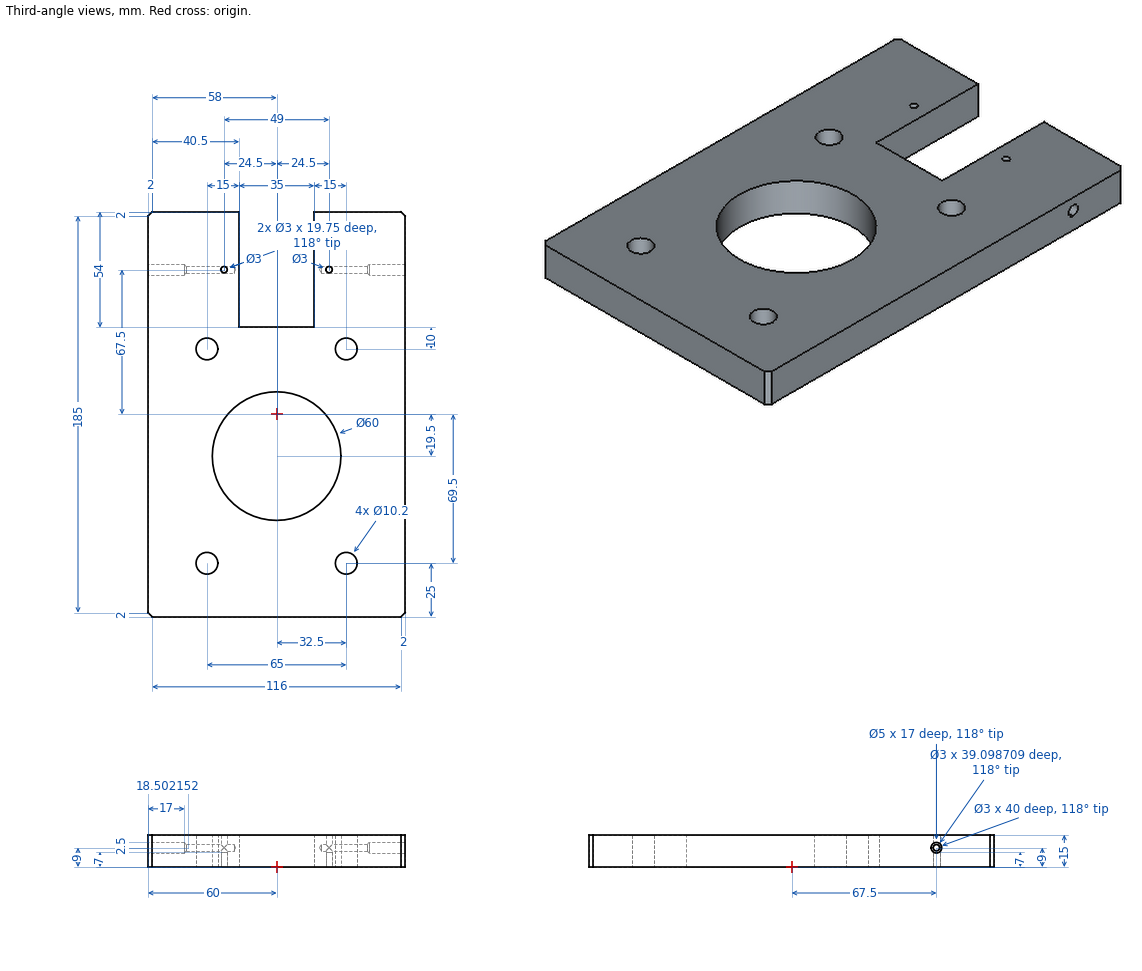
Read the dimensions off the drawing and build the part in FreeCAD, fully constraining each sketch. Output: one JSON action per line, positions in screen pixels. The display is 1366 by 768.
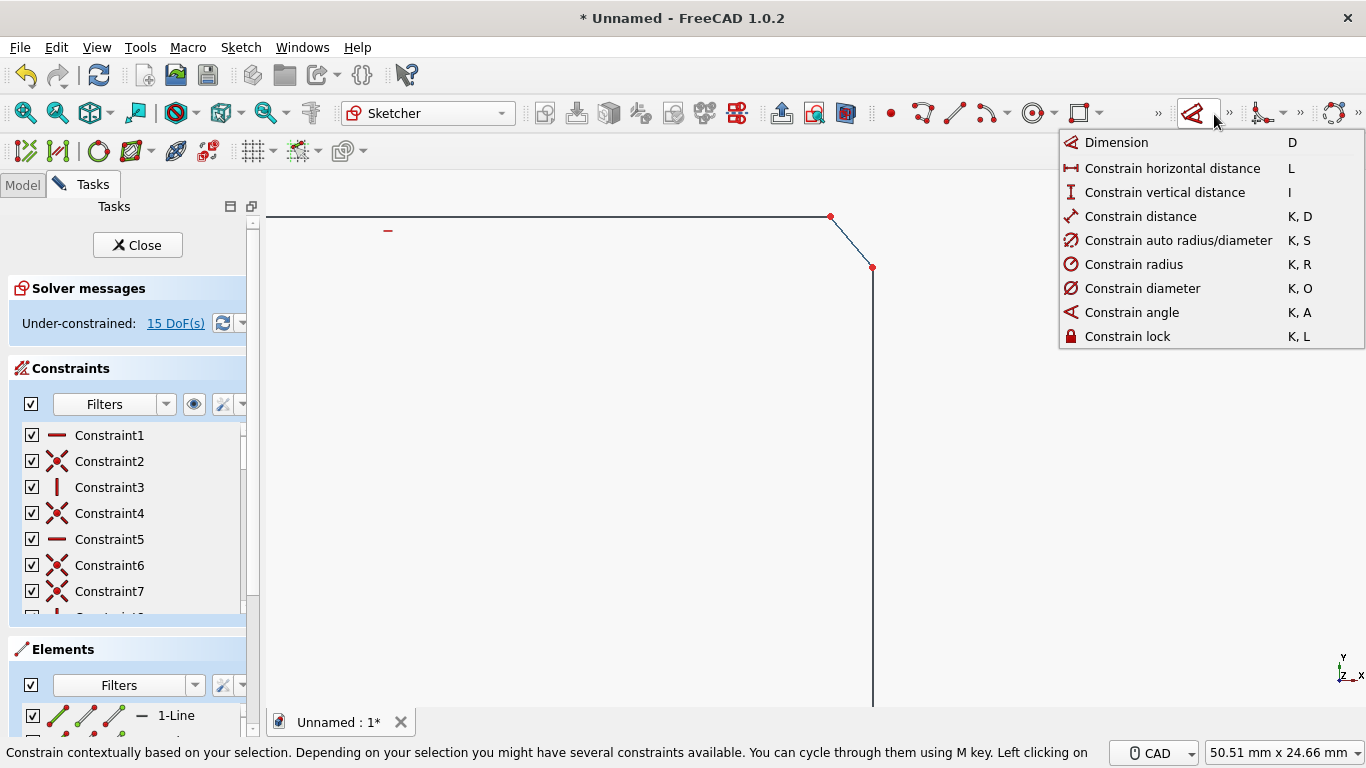
{"action": "left_click", "coordinate": [1212, 168]}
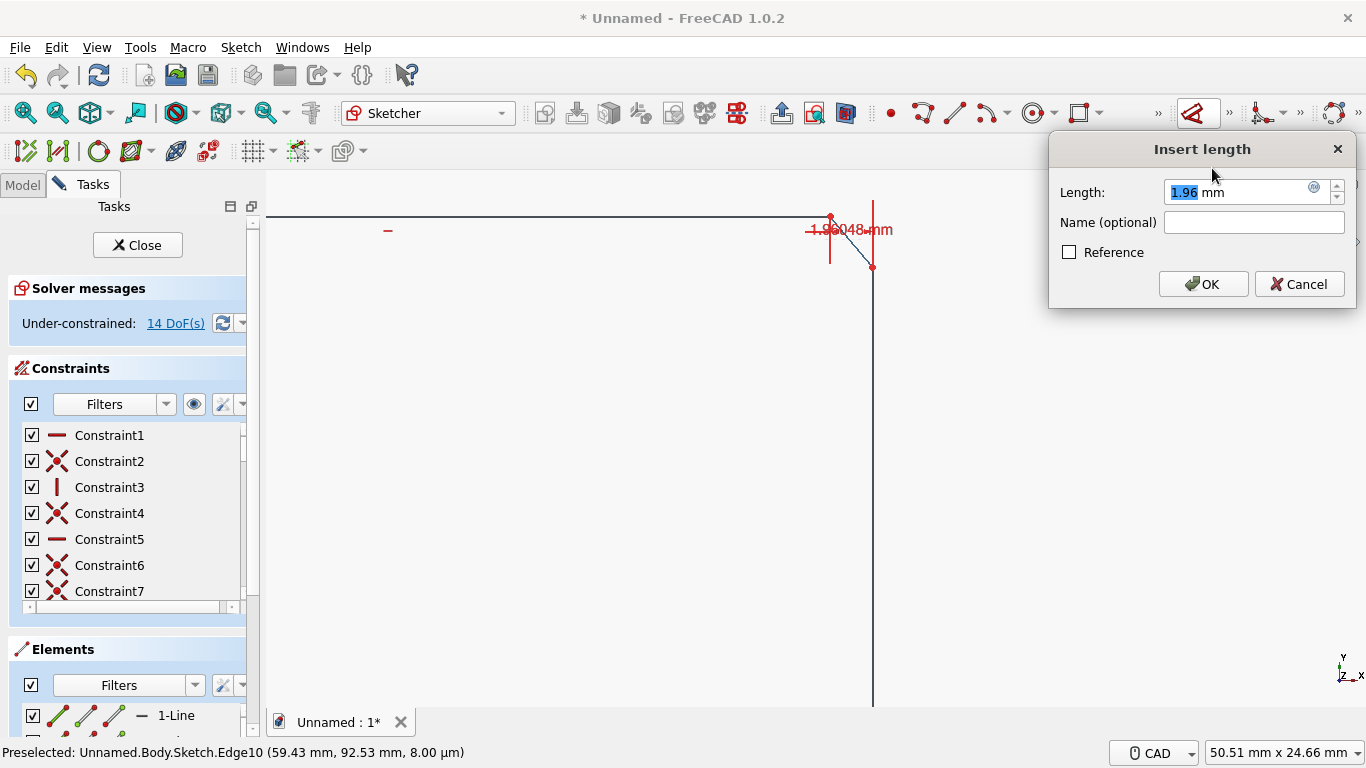
{"action": "type", "text": "2"}
{"action": "key", "text": "Return"}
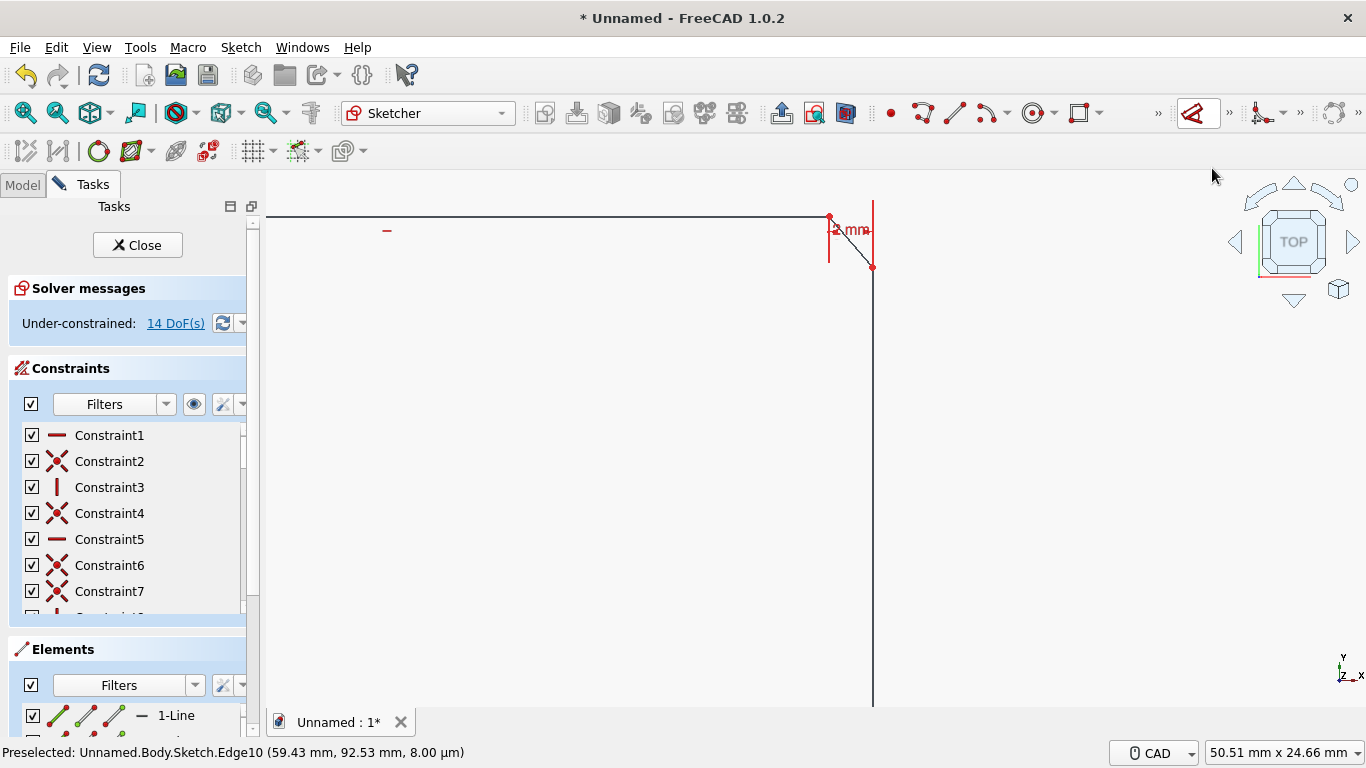
{"action": "left_click", "coordinate": [860, 252]}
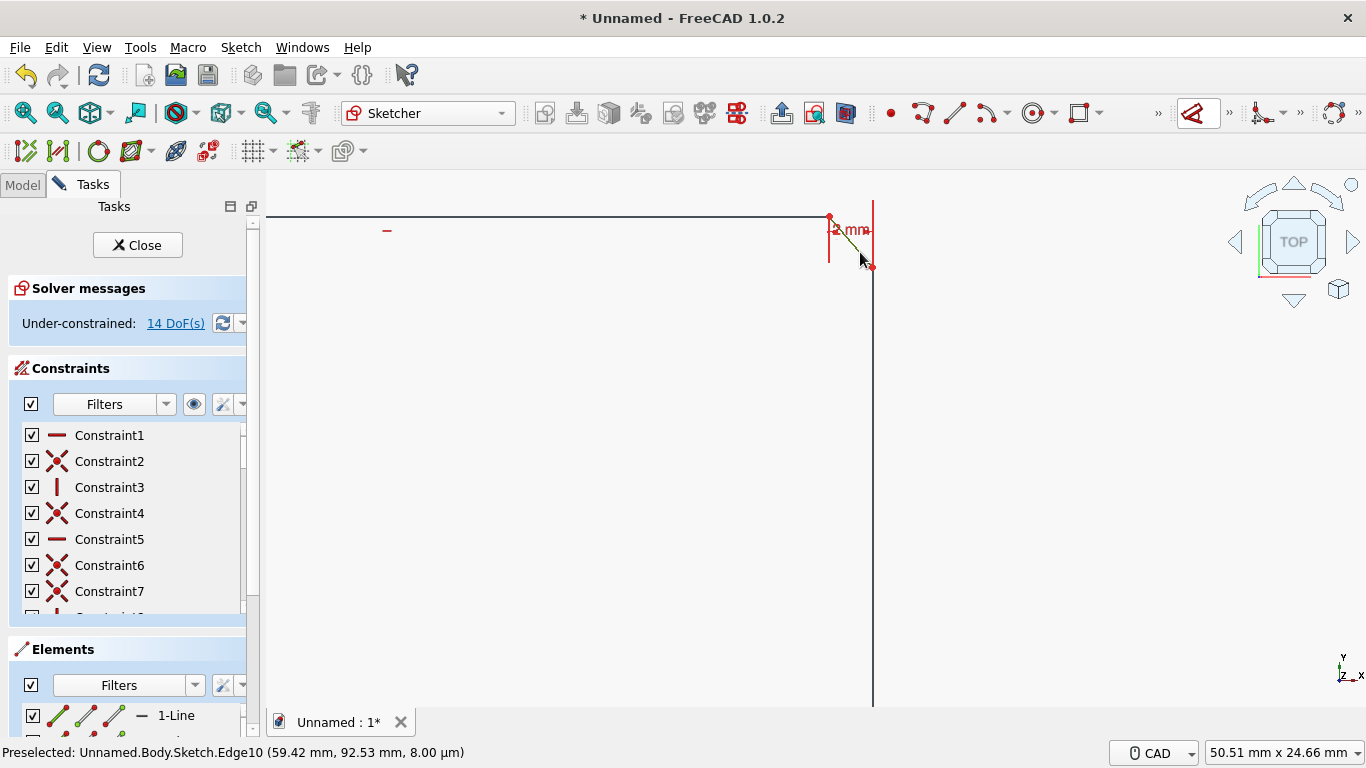
{"action": "left_click", "coordinate": [1214, 114]}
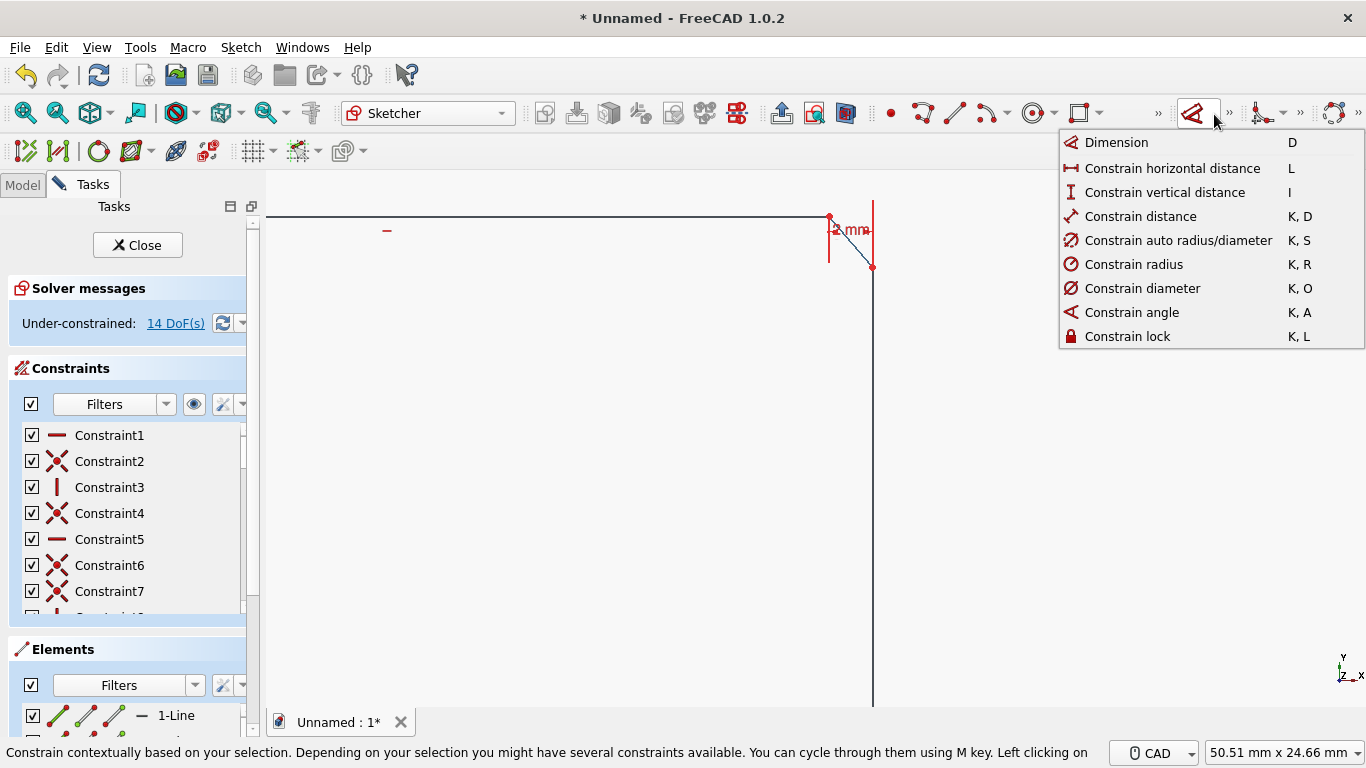
{"action": "left_click", "coordinate": [1212, 192]}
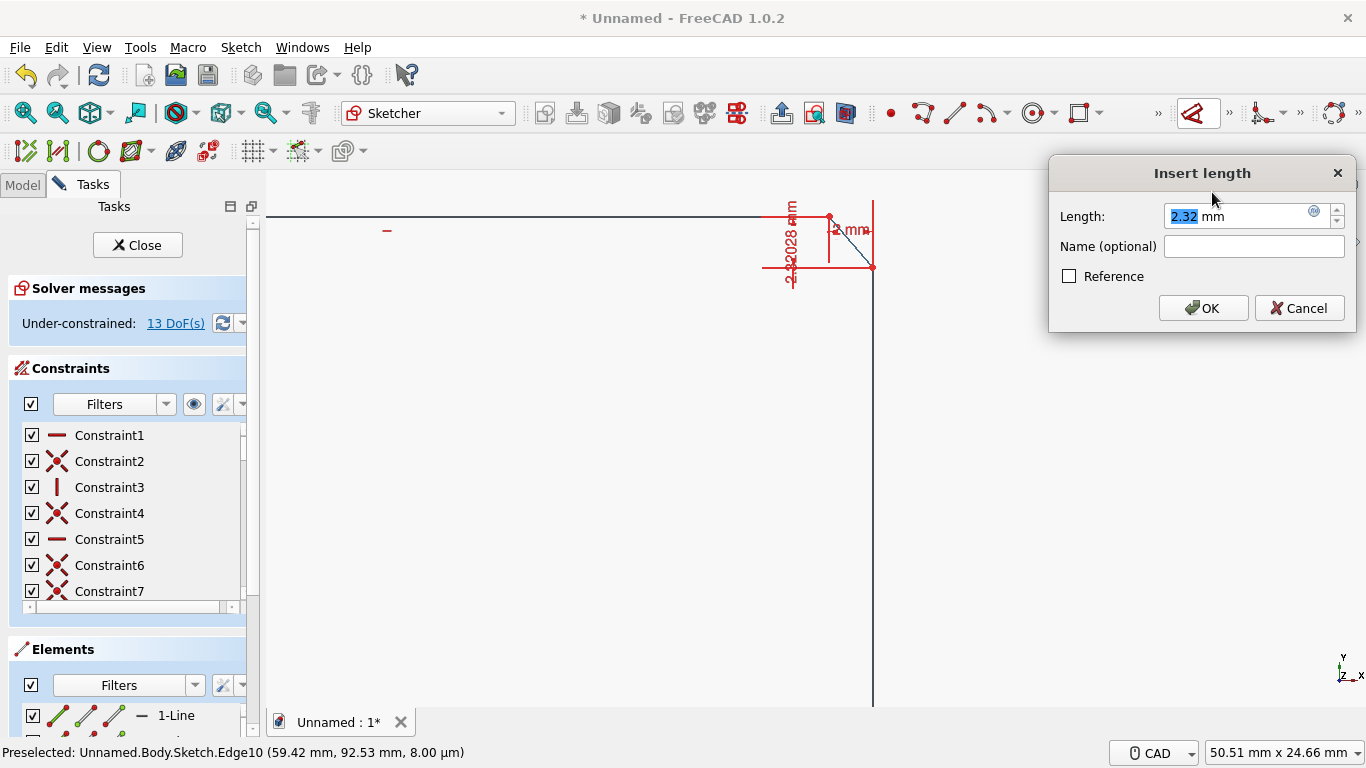
{"action": "type", "text": "2"}
{"action": "key", "text": "Return"}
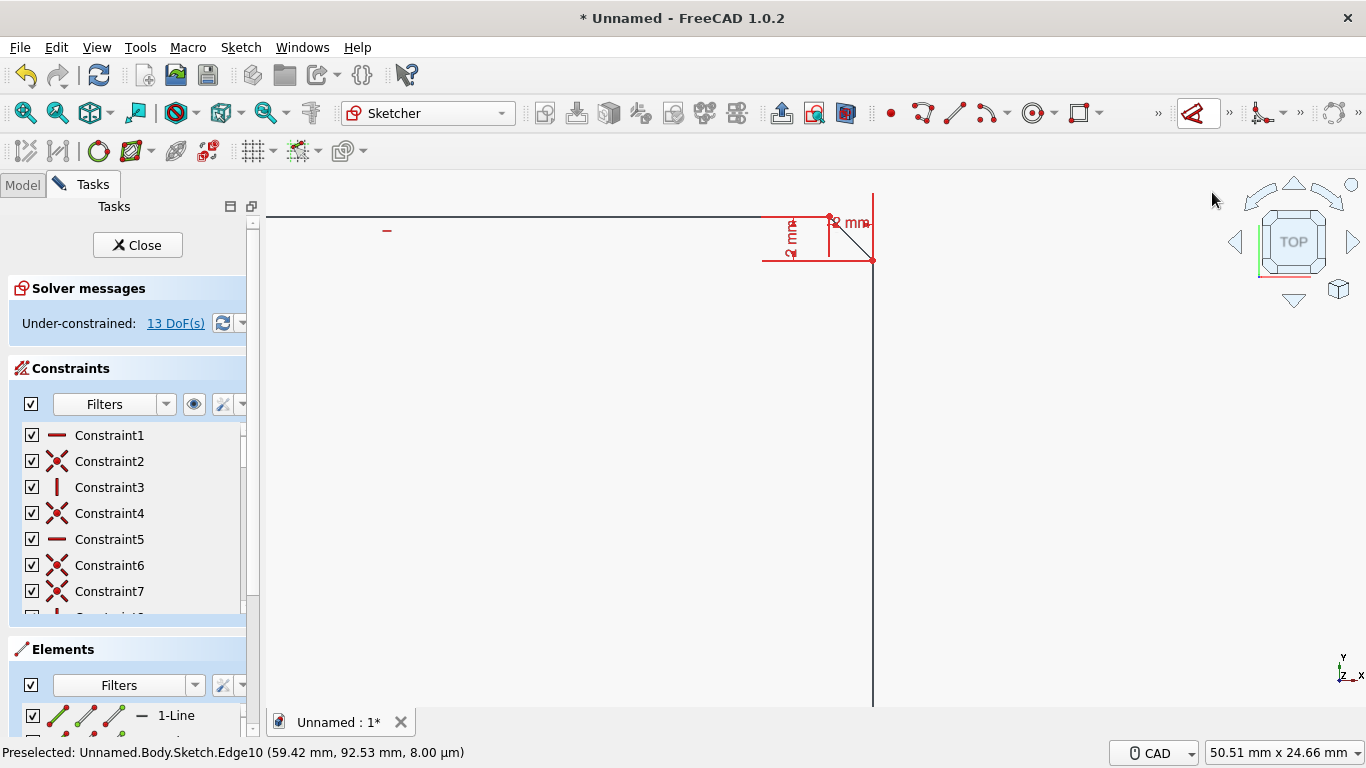
{"action": "scroll", "coordinate": [865, 256], "scroll_direction": "down", "scroll_amount": 12}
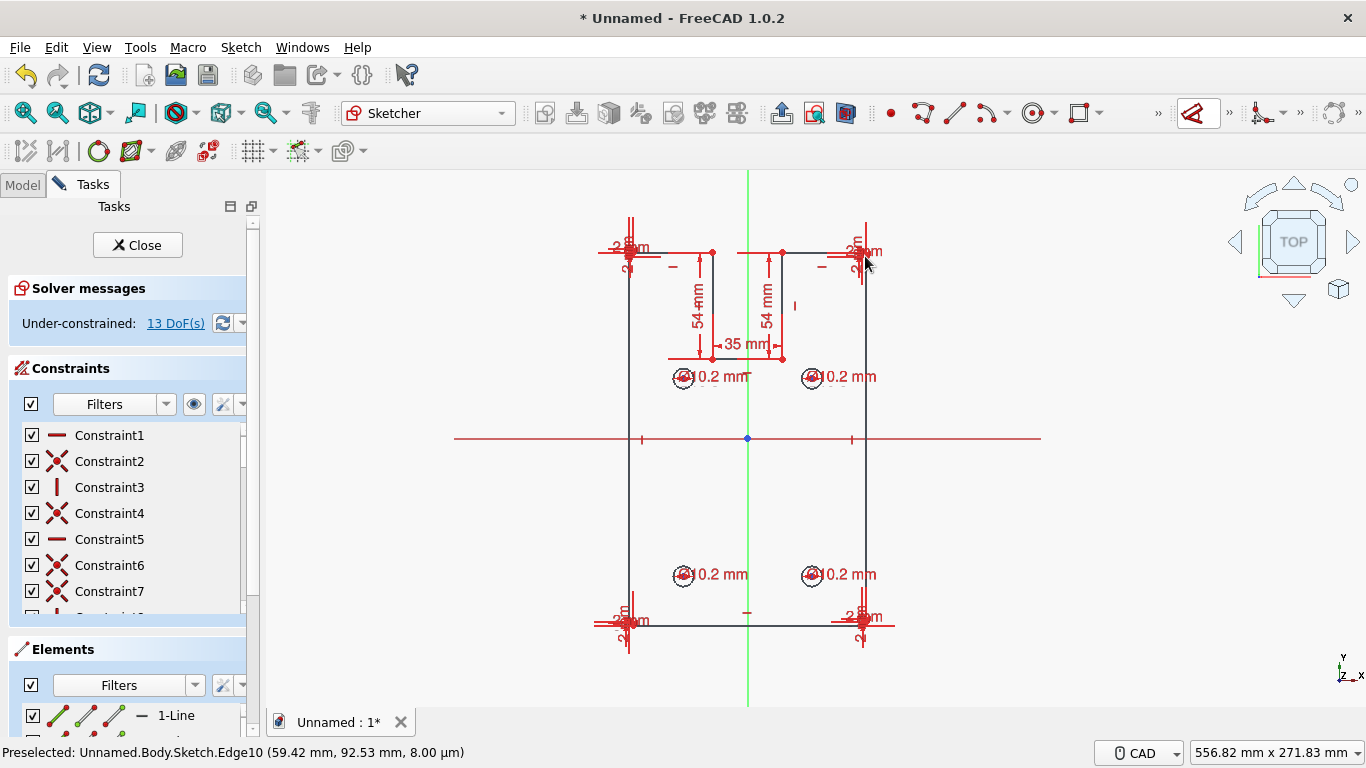
{"action": "left_click", "coordinate": [629, 366]}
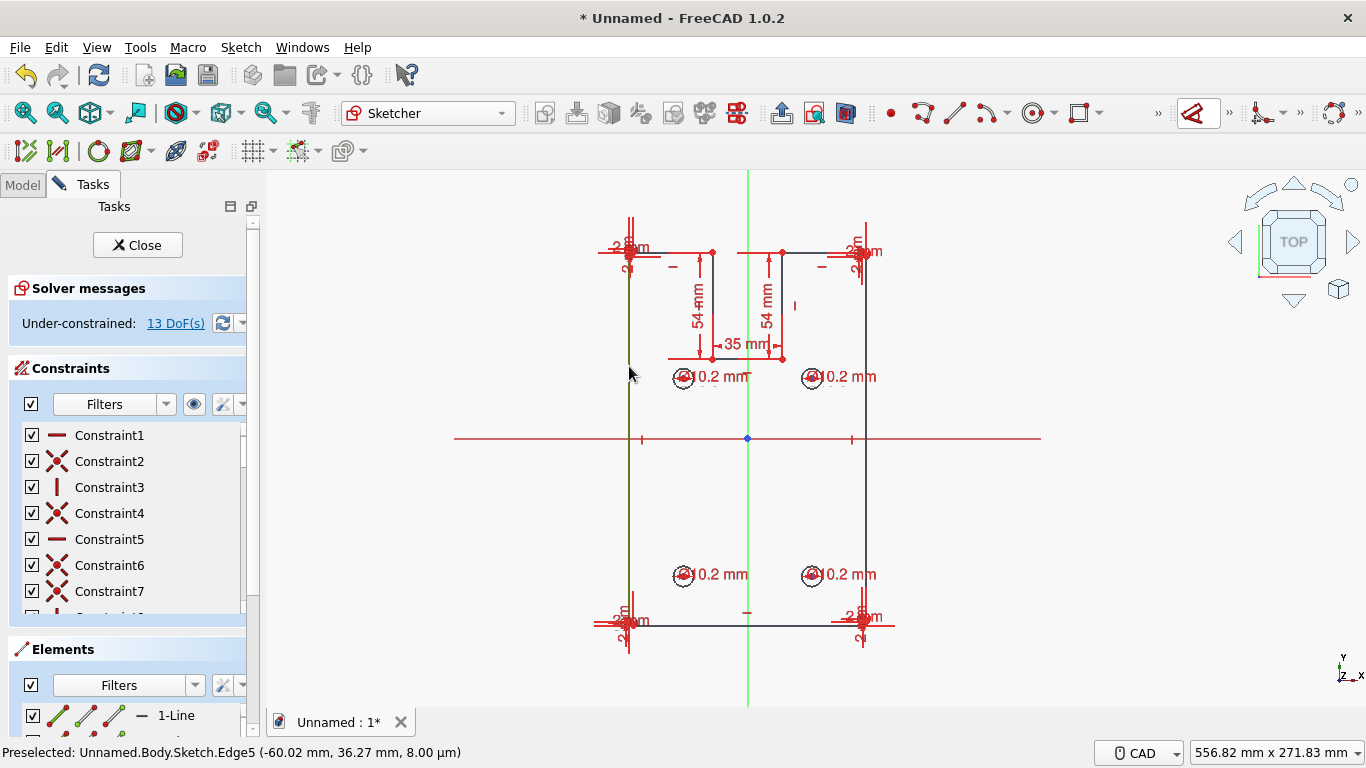
{"action": "key", "text": "i"}